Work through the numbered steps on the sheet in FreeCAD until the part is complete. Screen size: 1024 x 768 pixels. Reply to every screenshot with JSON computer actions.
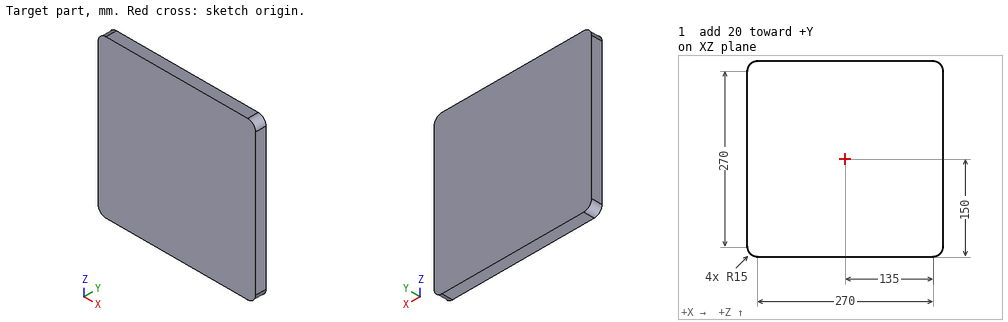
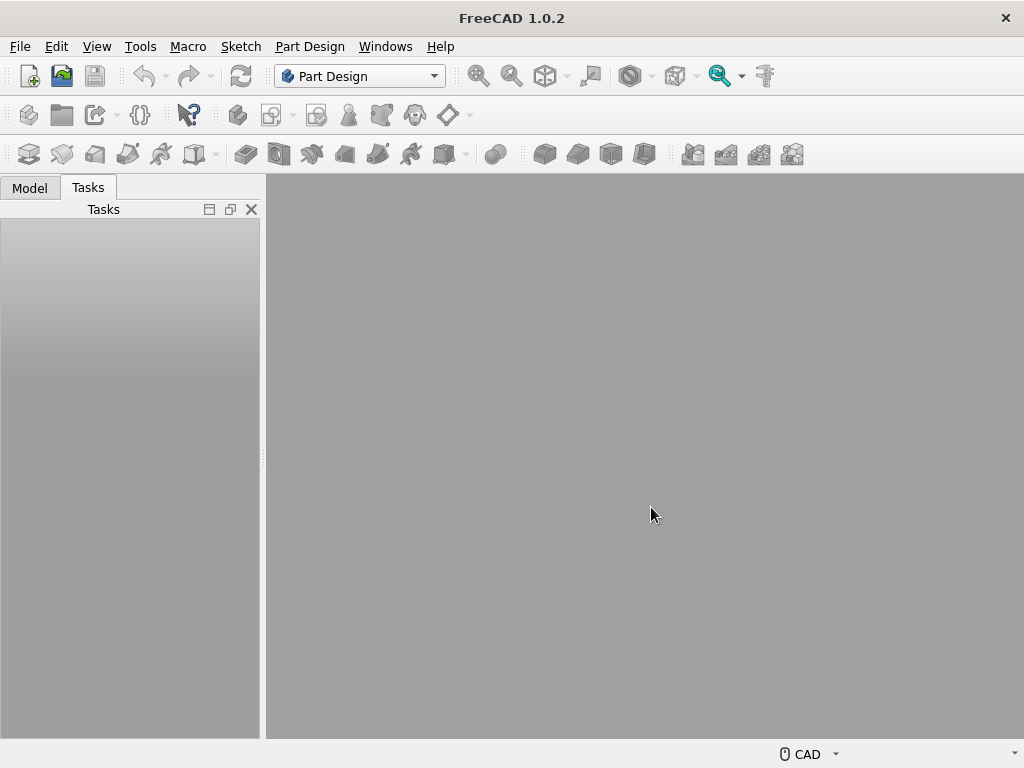
{"action": "left_click", "coordinate": [29, 76]}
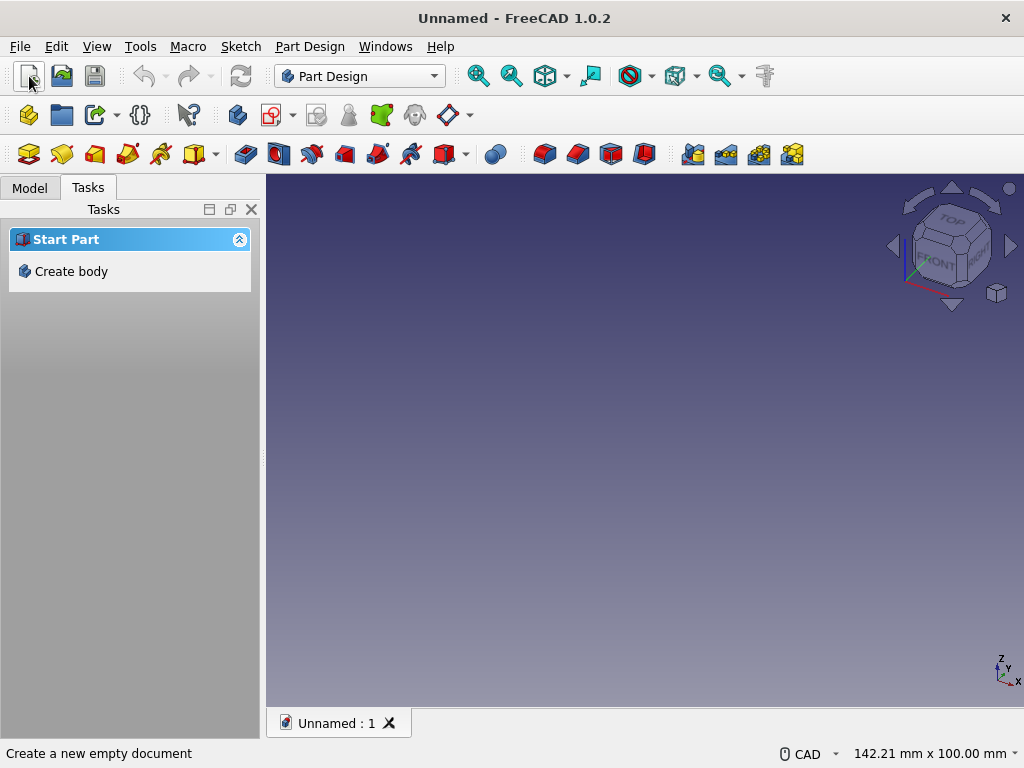
{"action": "left_click", "coordinate": [270, 116]}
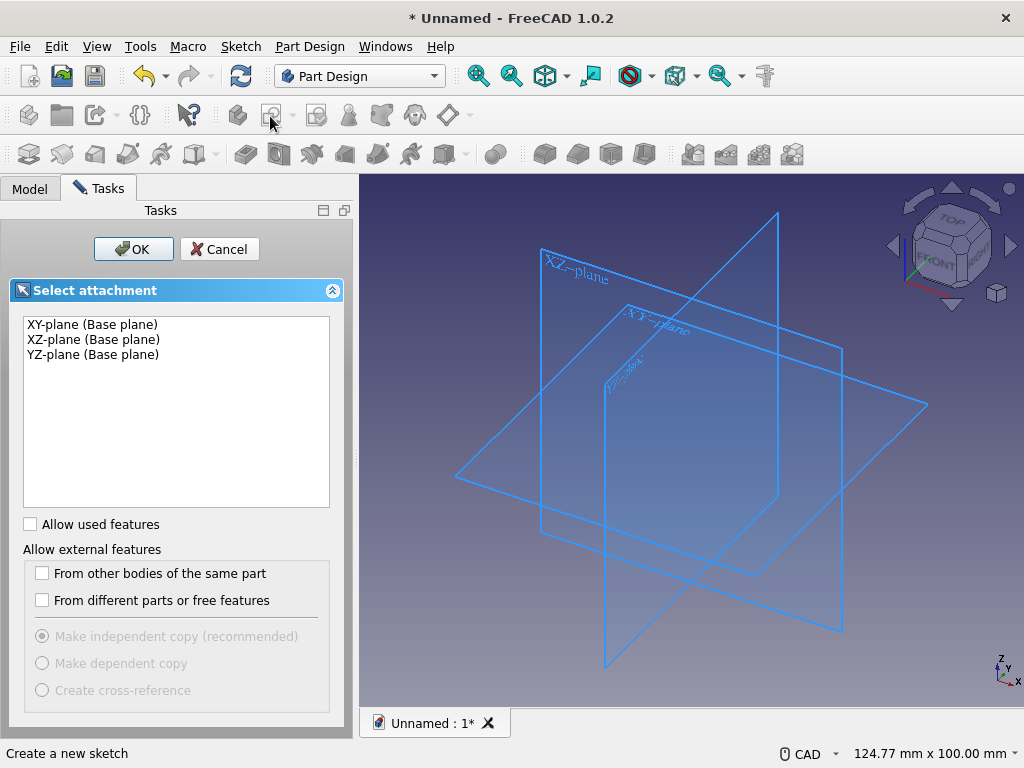
{"action": "left_click", "coordinate": [84, 340]}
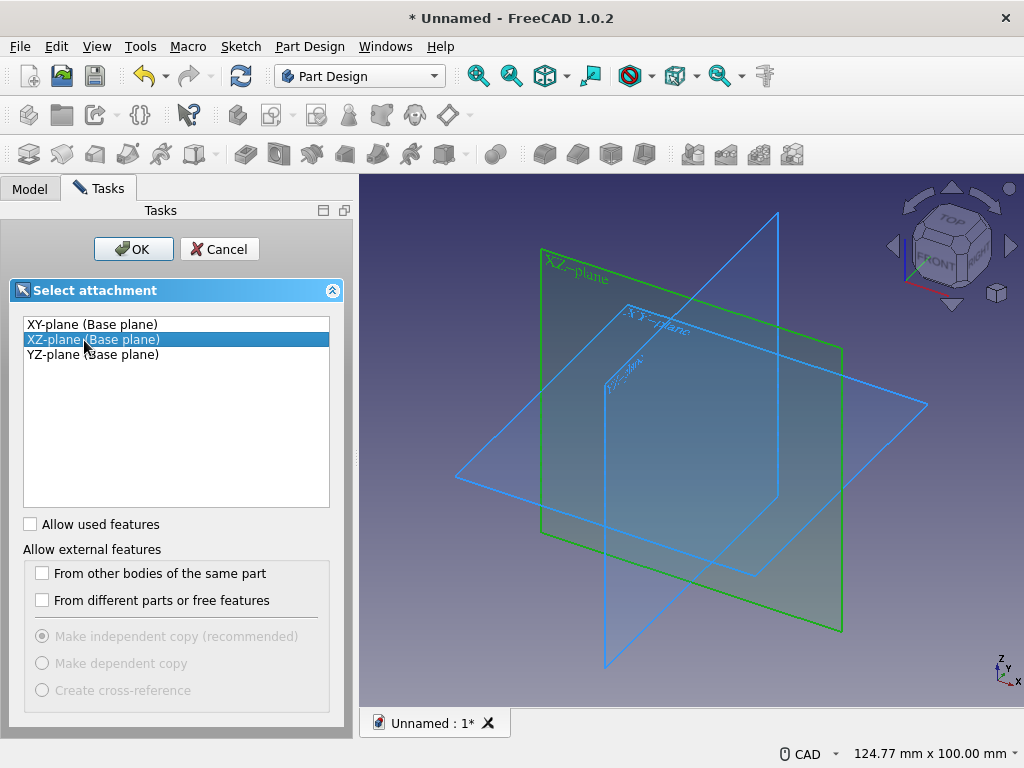
{"action": "left_click", "coordinate": [134, 249]}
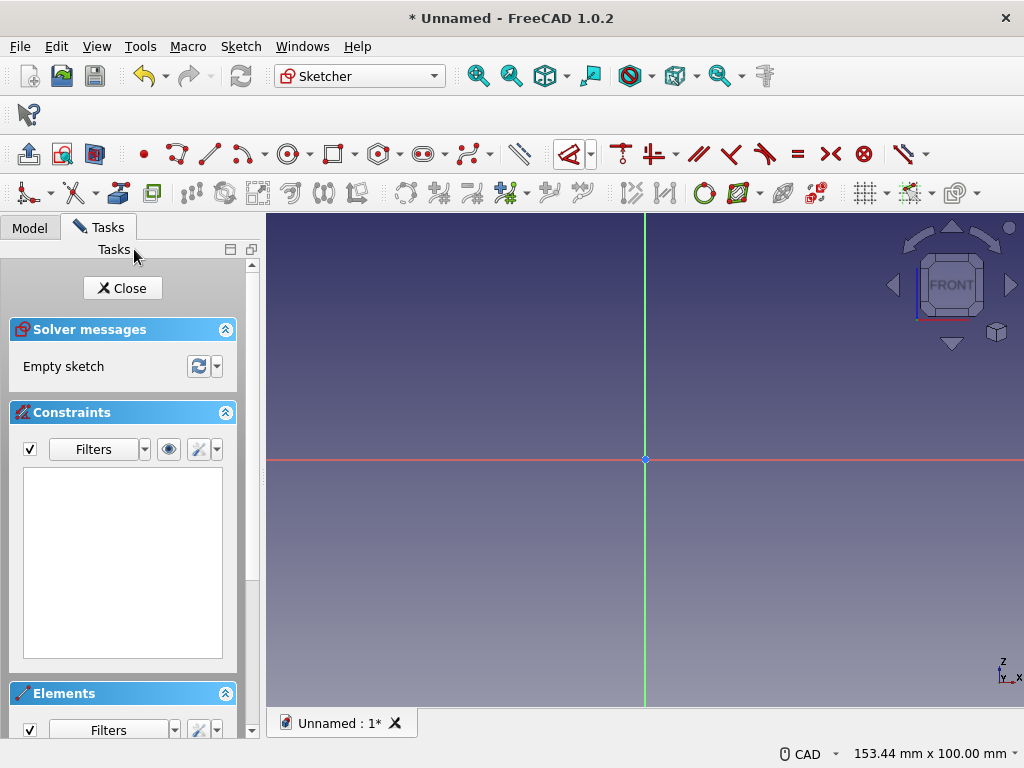
{"action": "scroll", "coordinate": [559, 460], "scroll_direction": "down", "scroll_amount": 8}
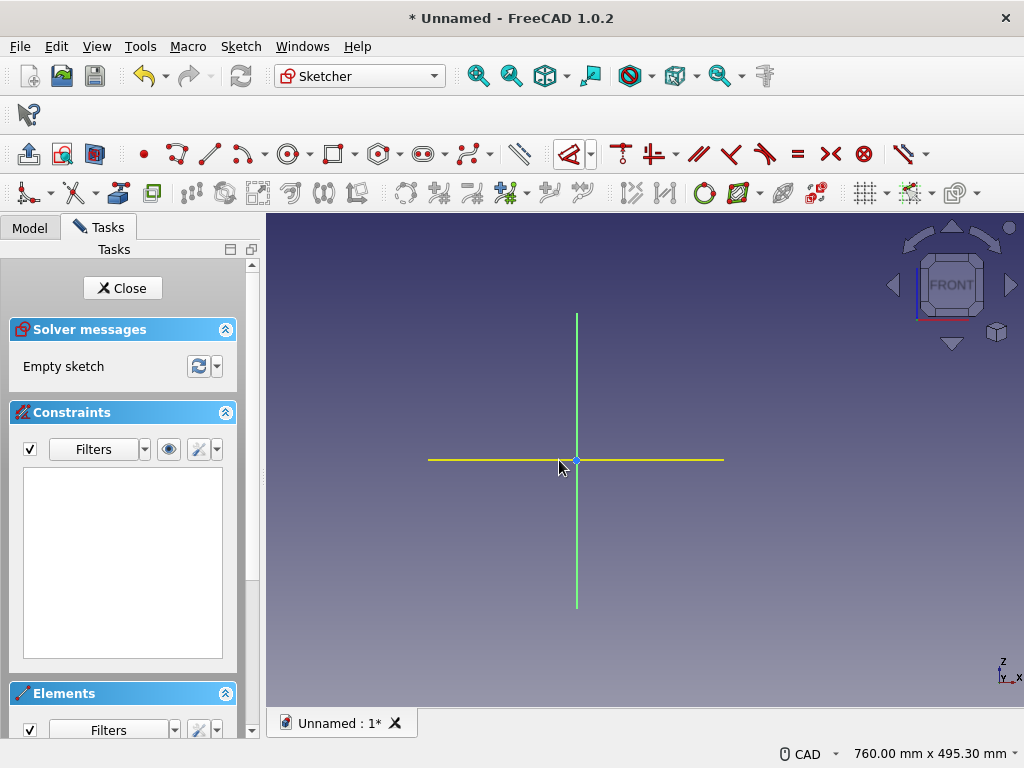
{"action": "left_click", "coordinate": [210, 154]}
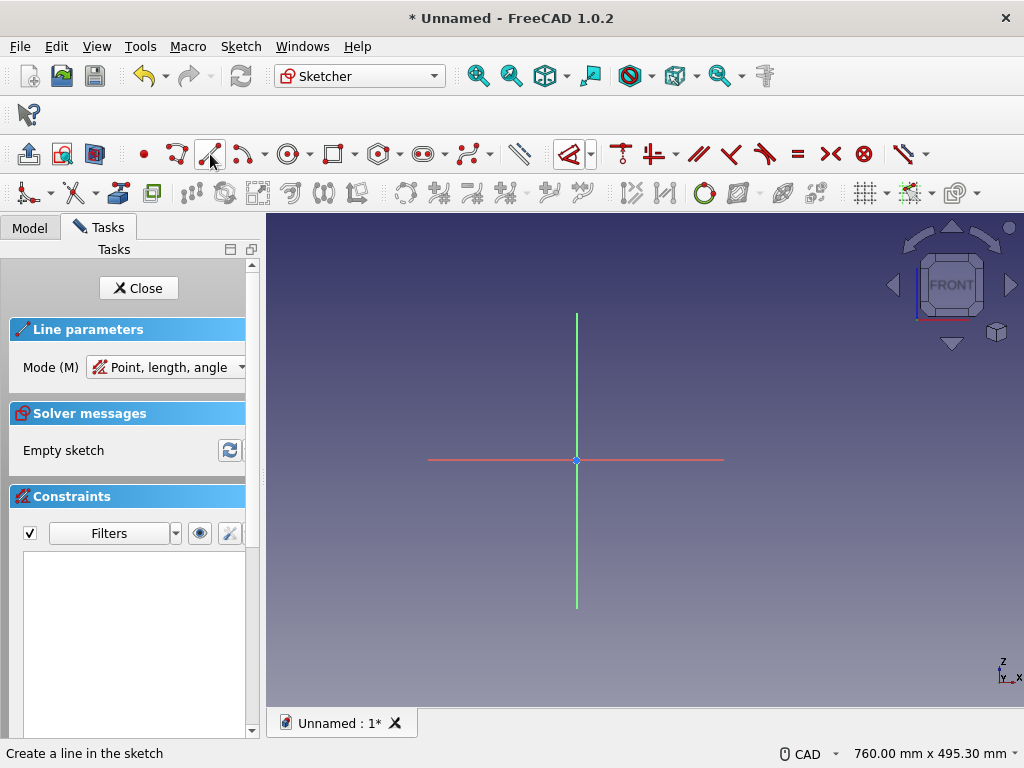
{"action": "left_click", "coordinate": [711, 610]}
{"action": "left_click", "coordinate": [442, 610]}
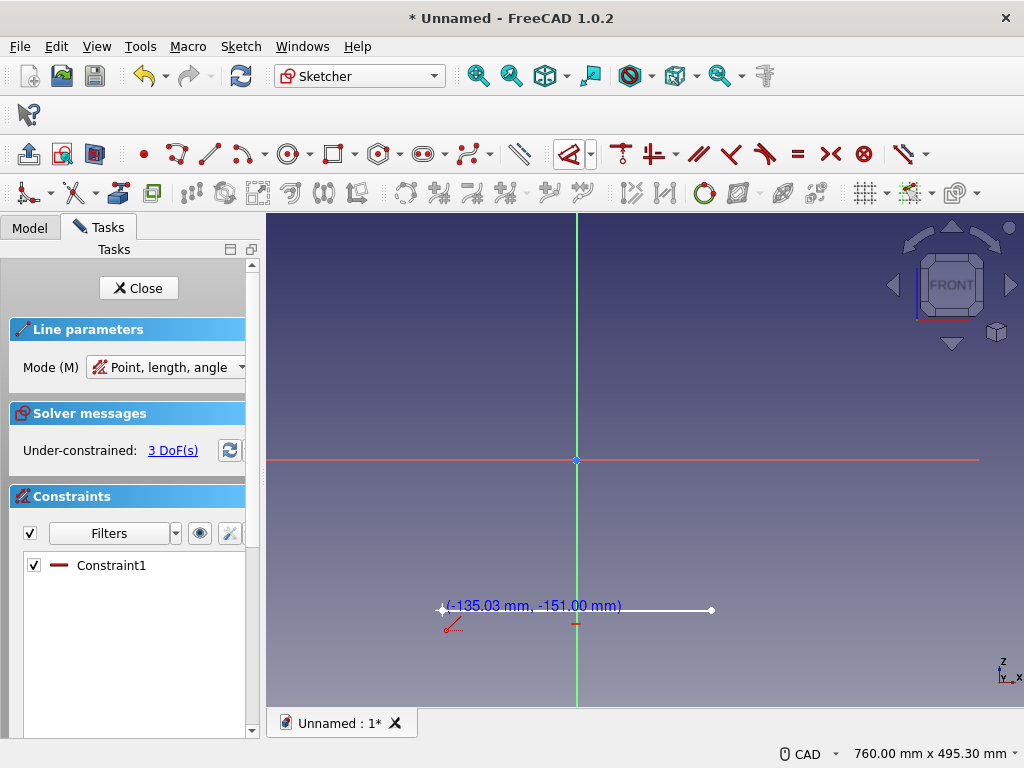
{"action": "left_click", "coordinate": [427, 595]}
{"action": "left_click", "coordinate": [427, 326]}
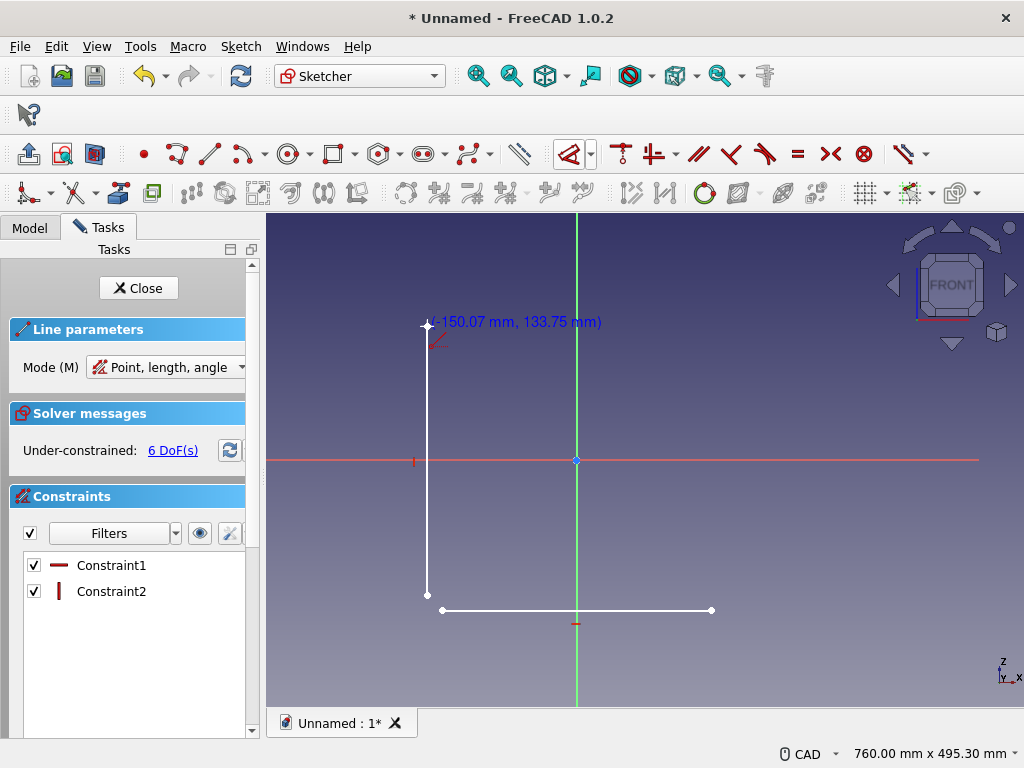
{"action": "left_click", "coordinate": [442, 311]}
{"action": "left_click", "coordinate": [711, 311]}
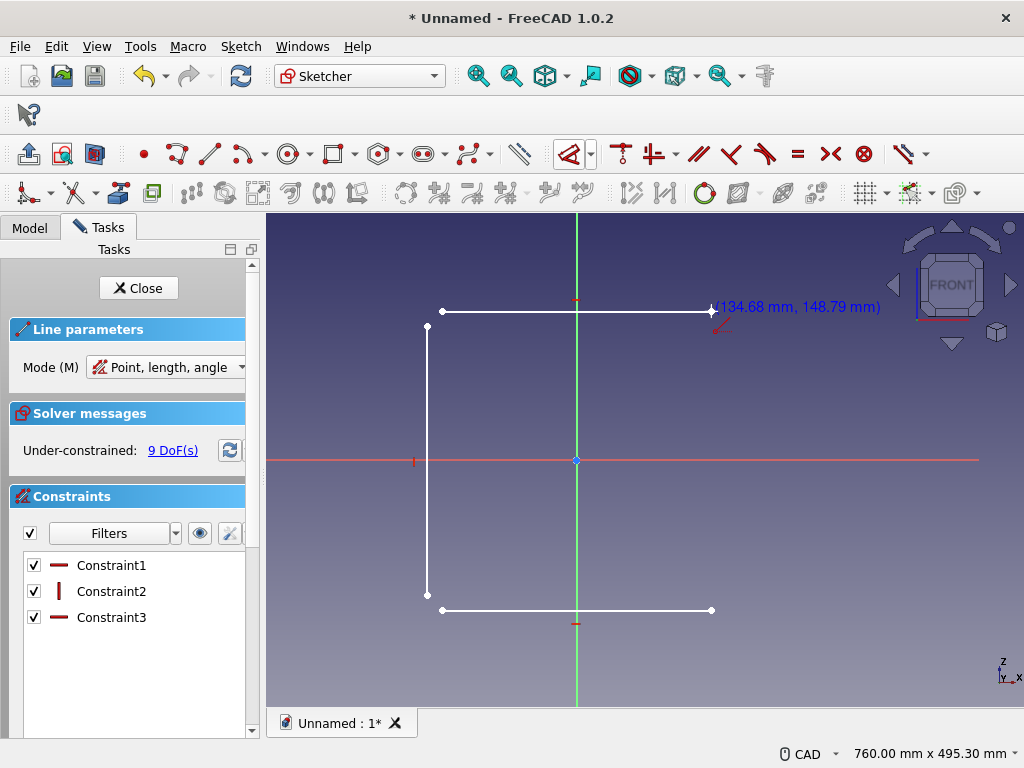
{"action": "left_click", "coordinate": [726, 326]}
{"action": "left_click", "coordinate": [726, 595]}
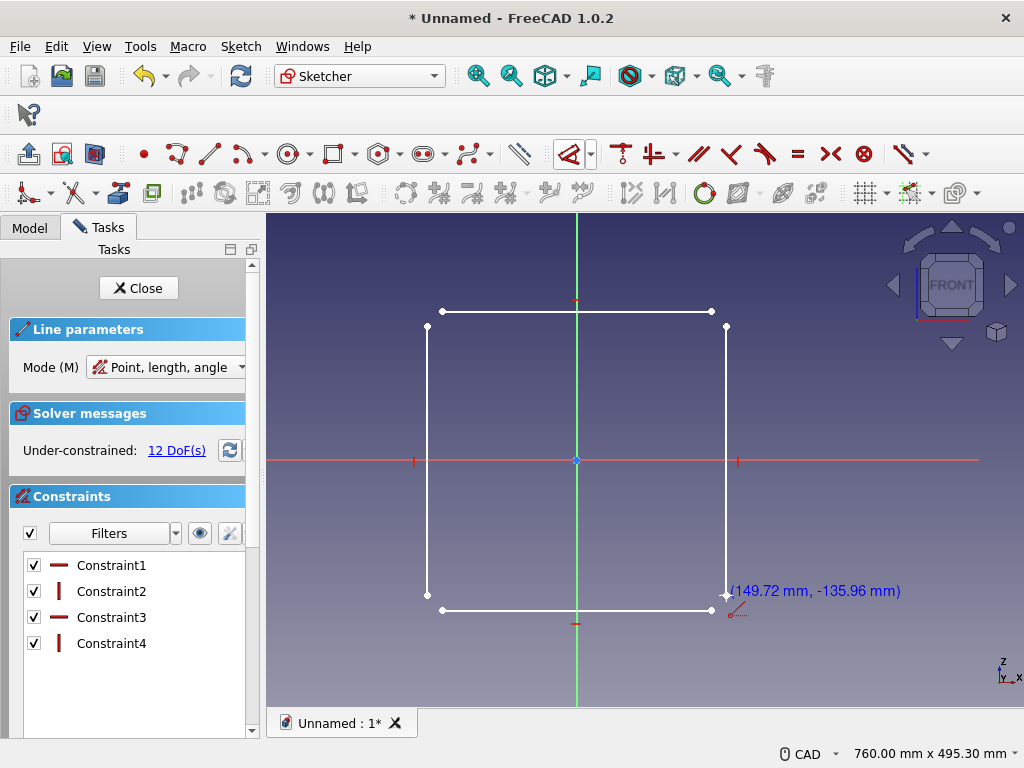
{"action": "left_click", "coordinate": [264, 154]}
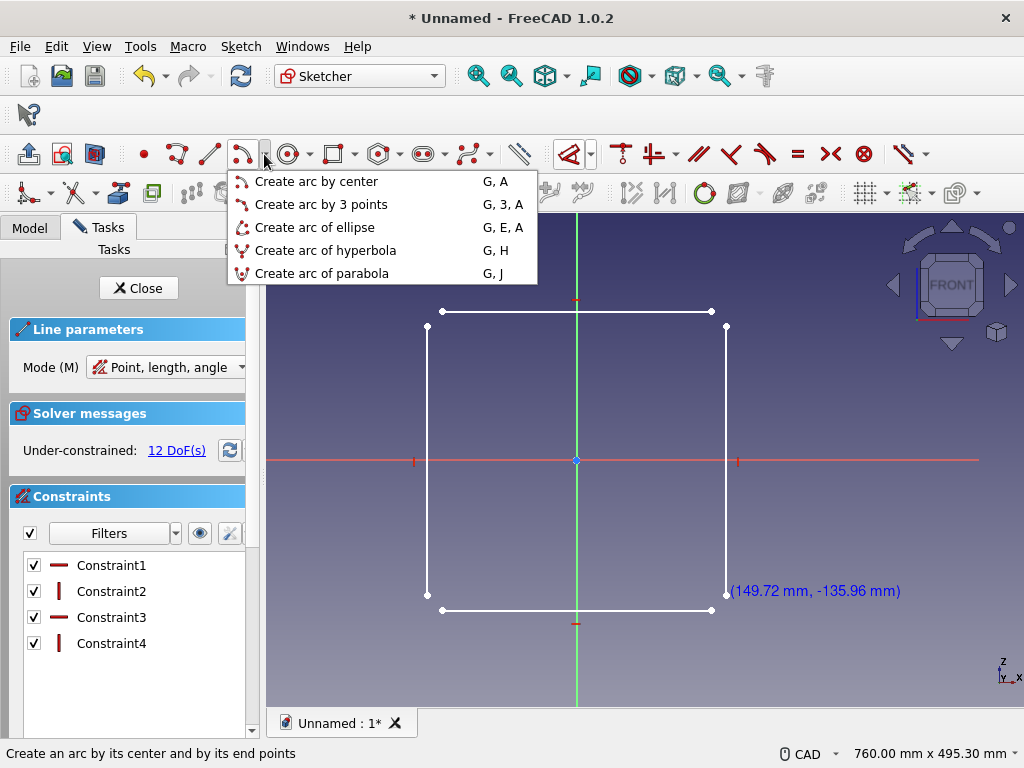
{"action": "left_click", "coordinate": [382, 204]}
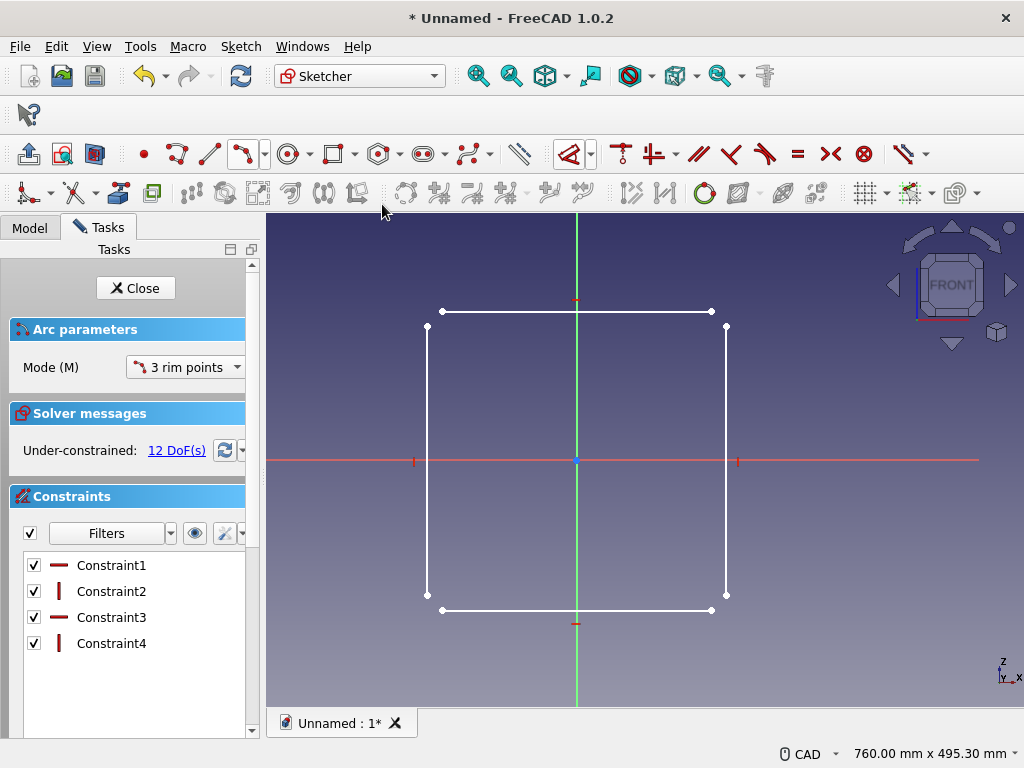
{"action": "left_click", "coordinate": [442, 611]}
{"action": "left_click", "coordinate": [427, 596]}